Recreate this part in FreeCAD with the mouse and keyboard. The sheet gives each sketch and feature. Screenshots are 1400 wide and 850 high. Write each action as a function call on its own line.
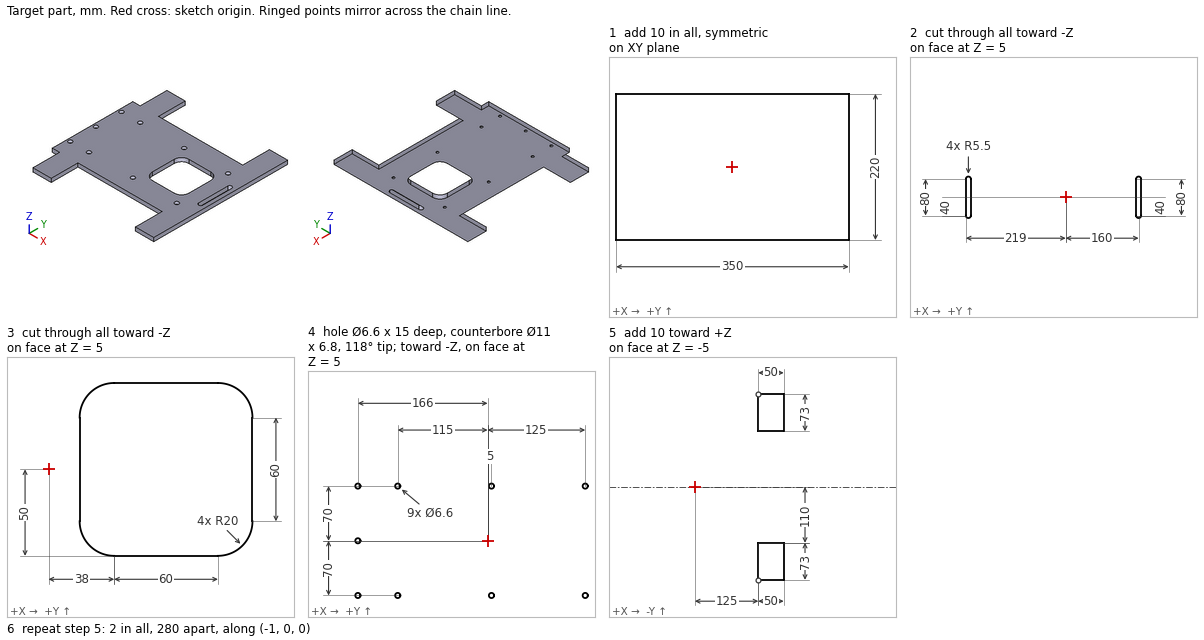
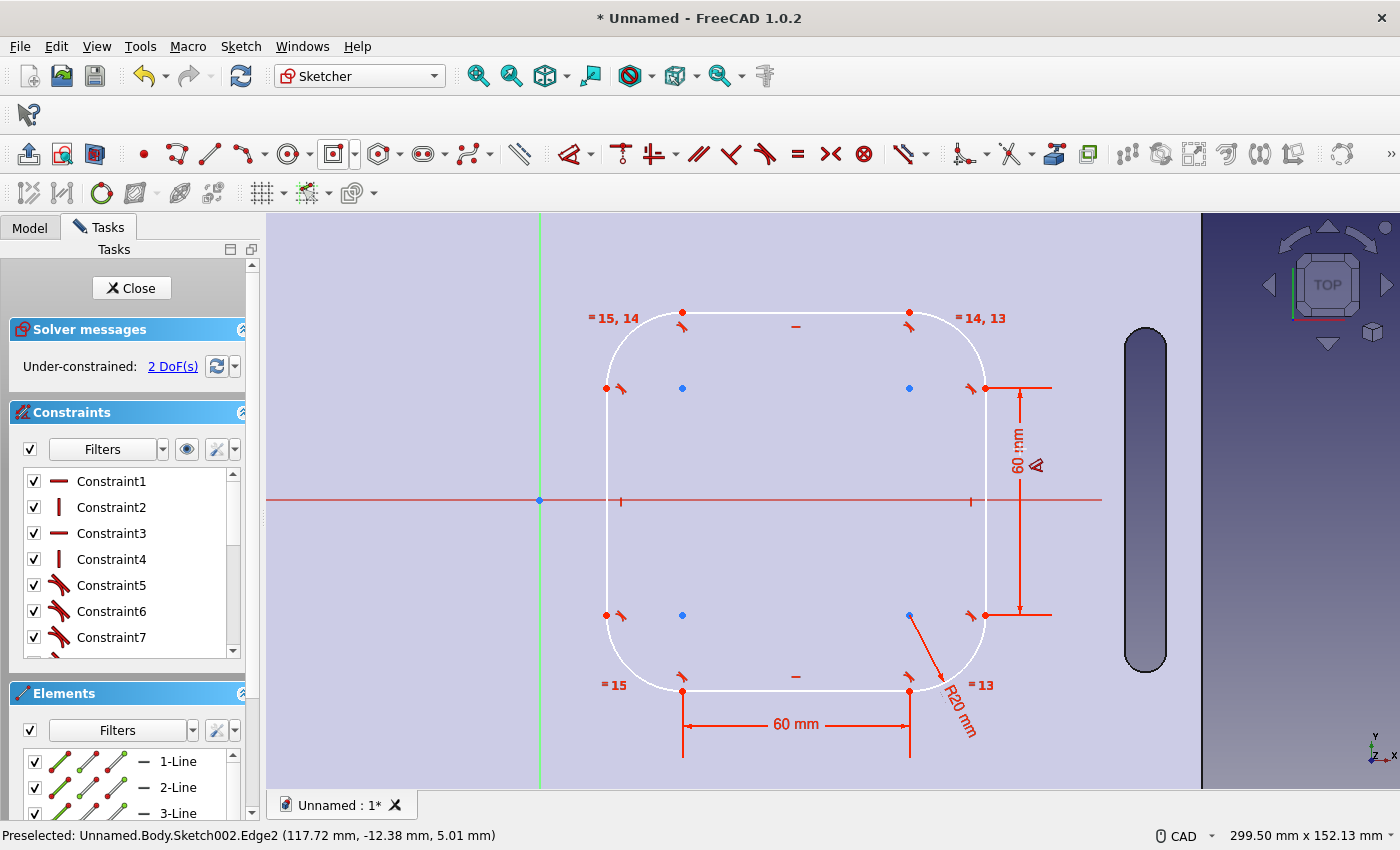
click(683, 691)
click(611, 725)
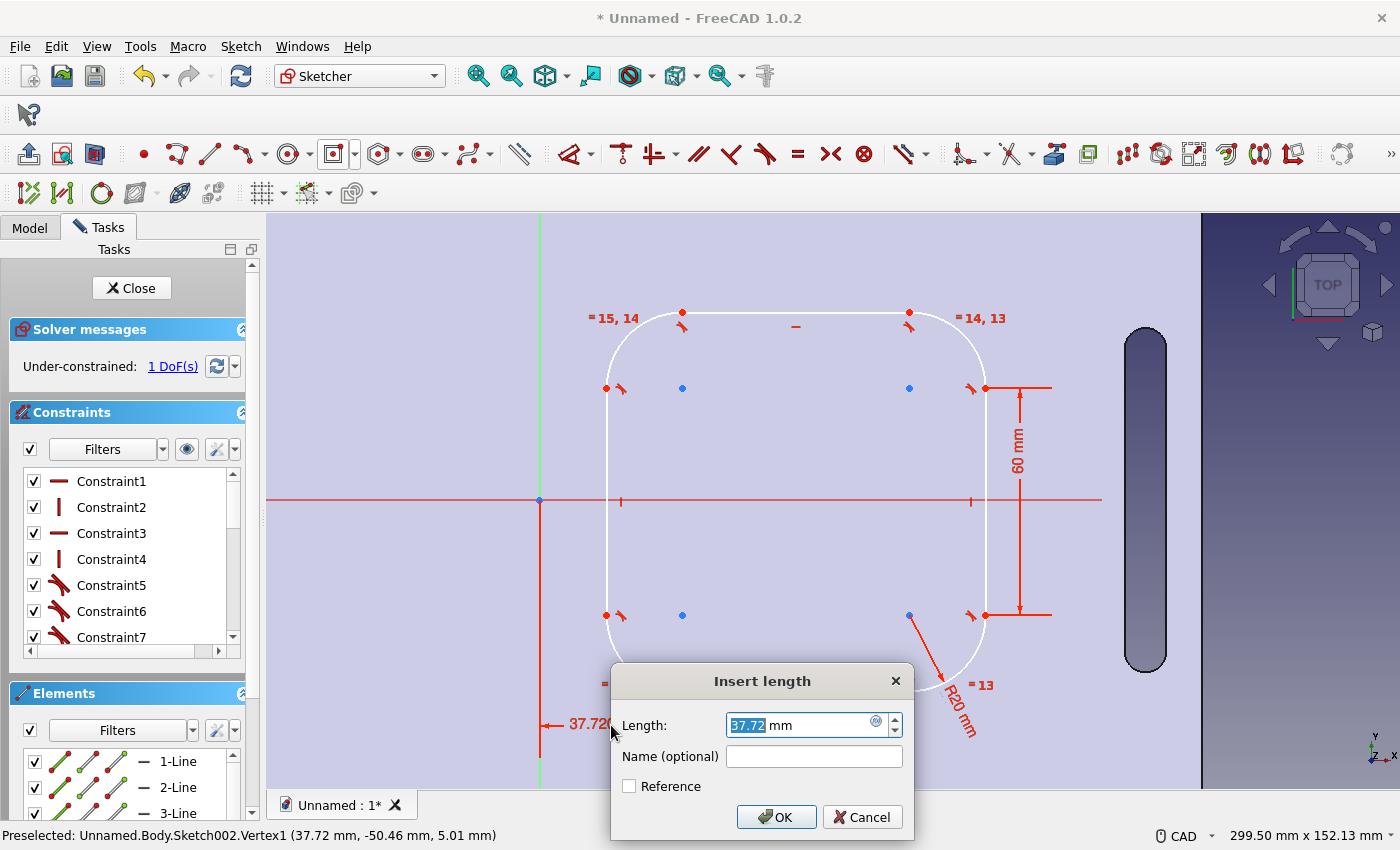
text(38)
key(Return)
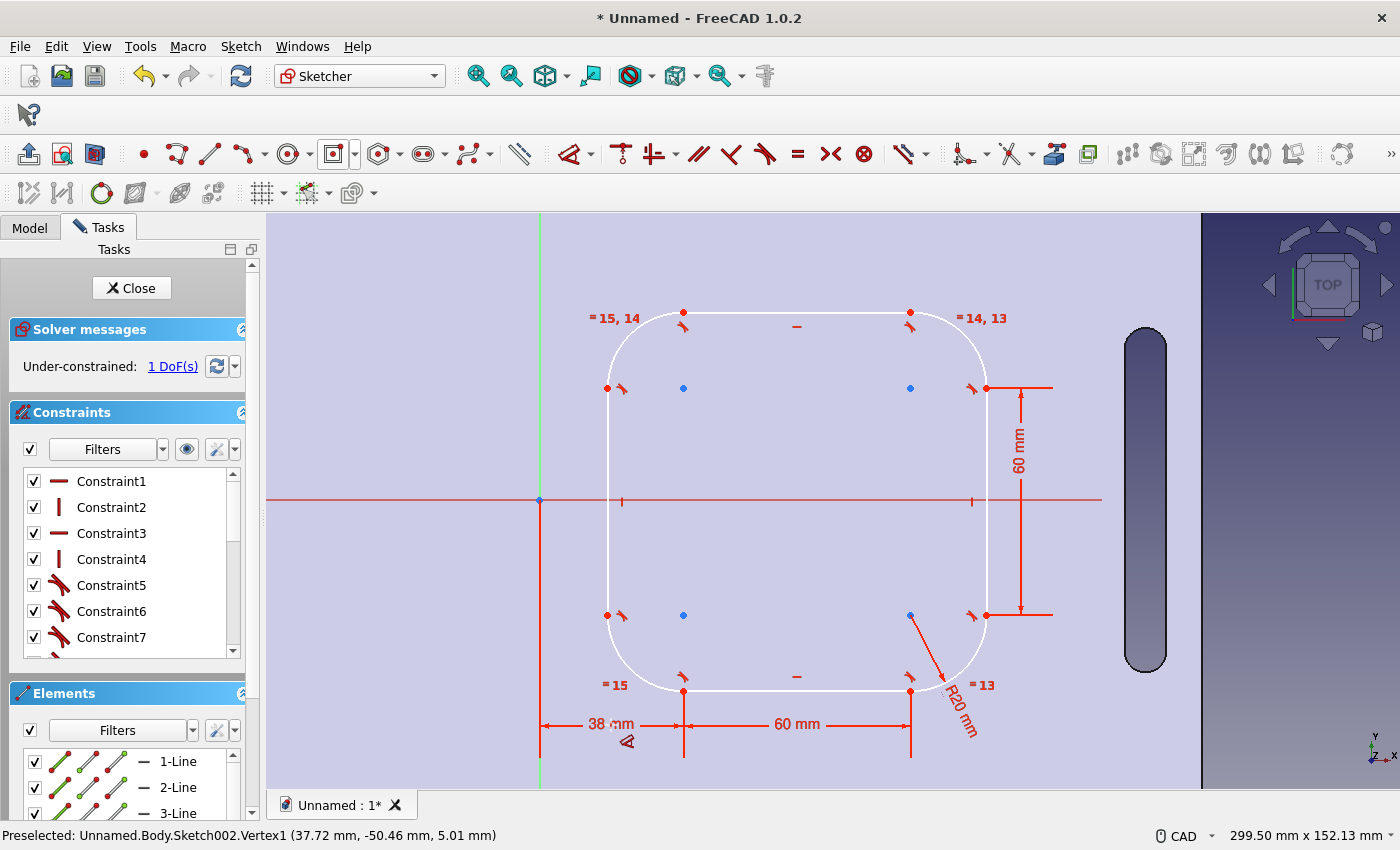
click(684, 691)
click(506, 596)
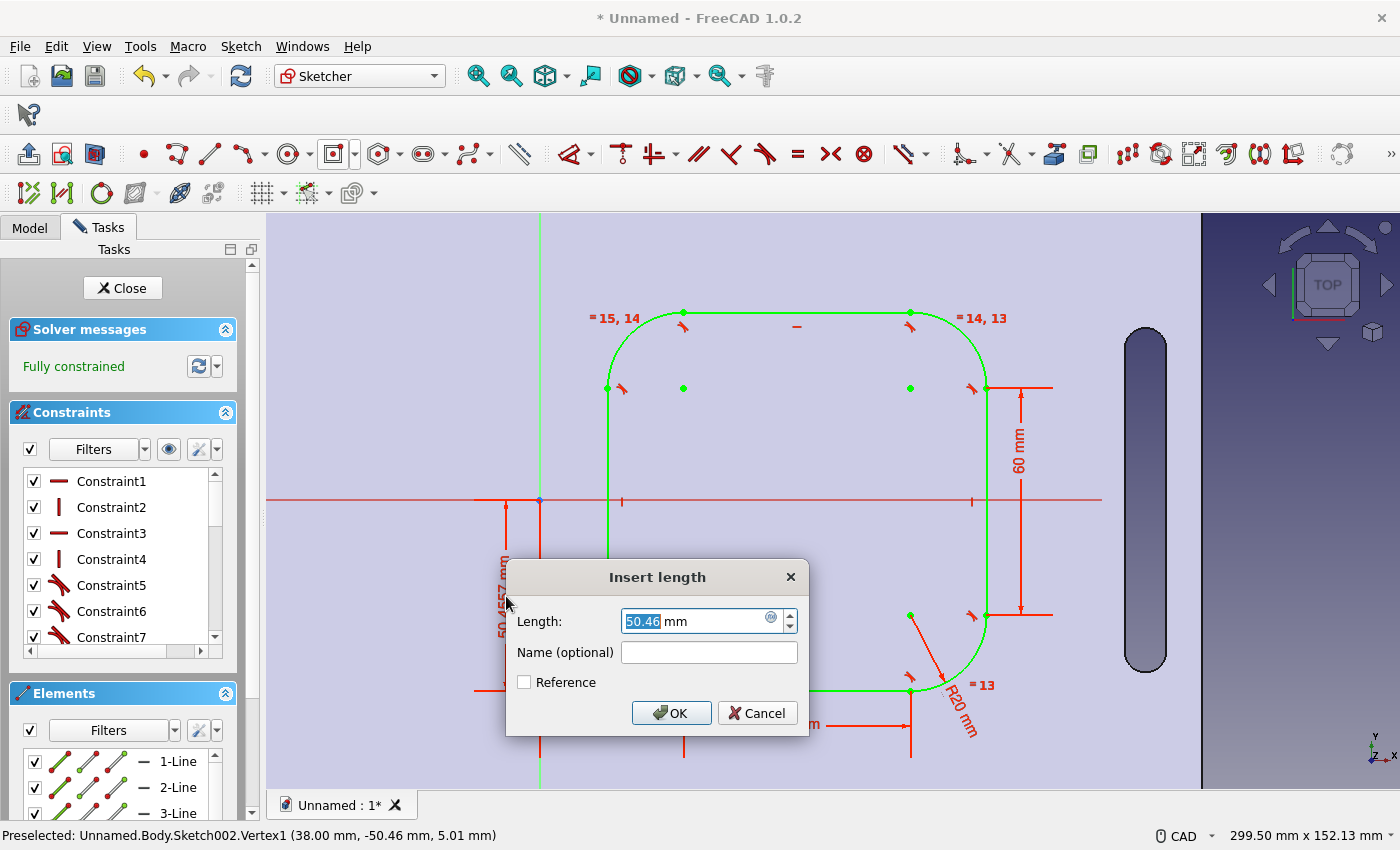
text(50)
key(Return)
key(Escape)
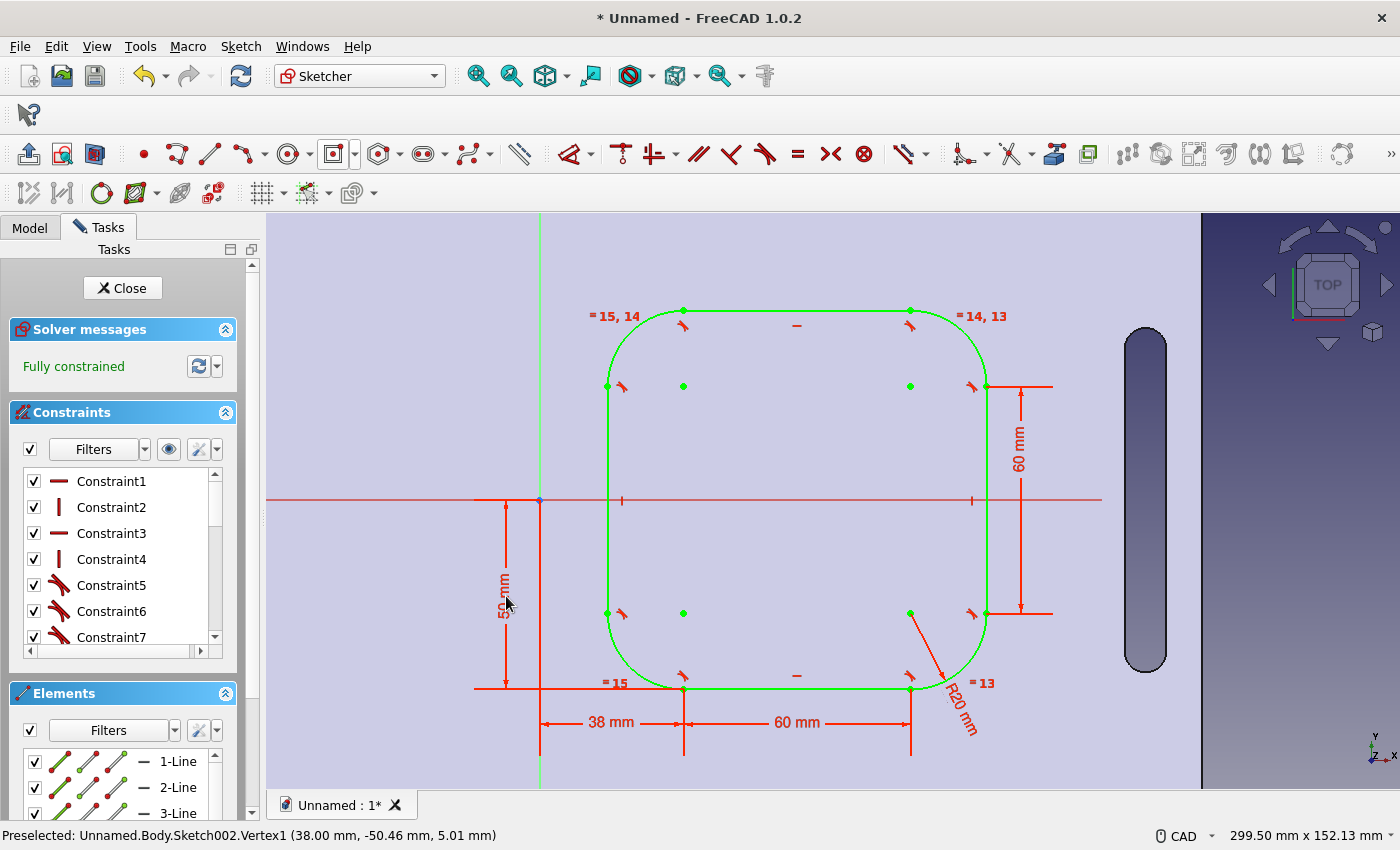
click(123, 288)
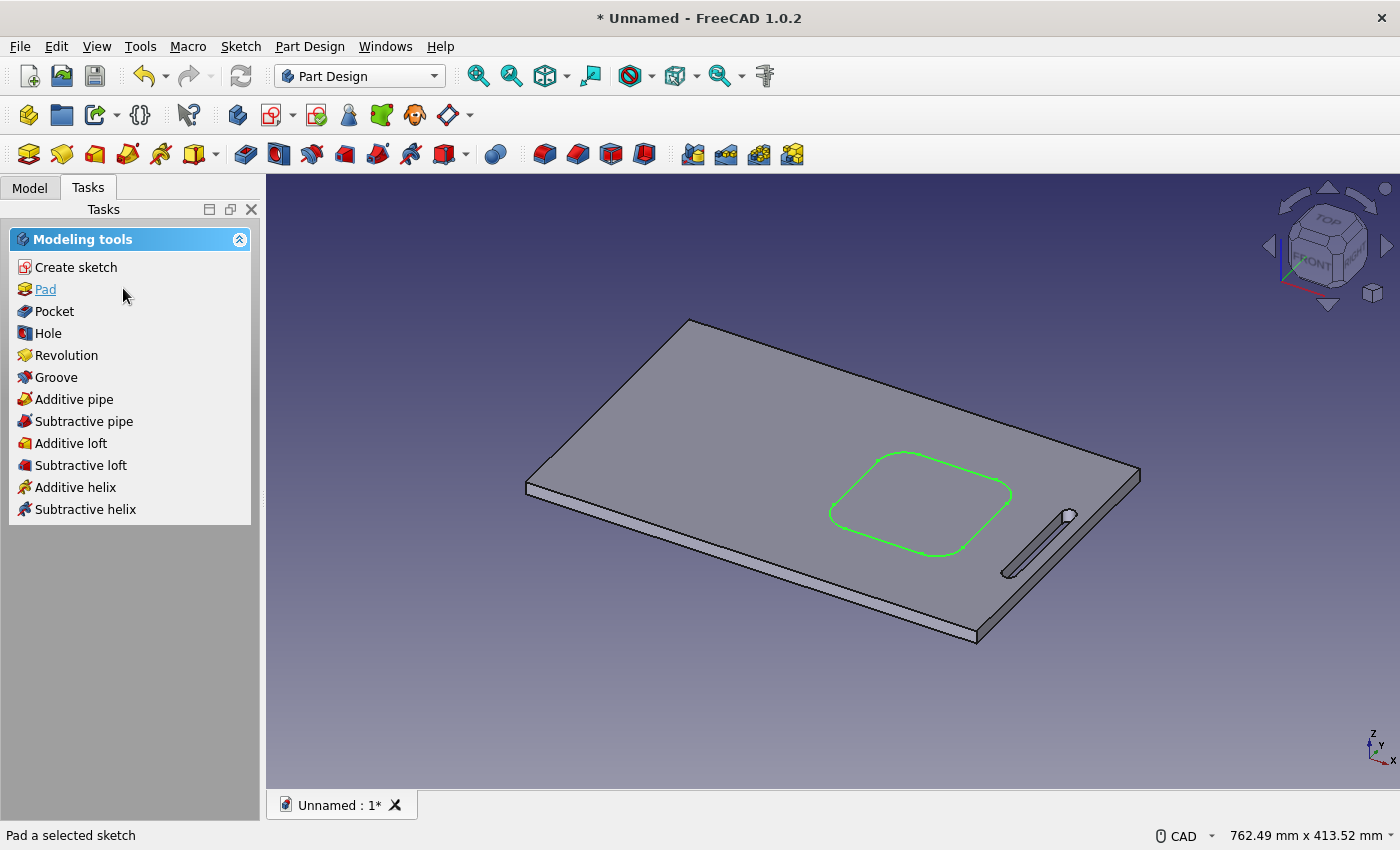
click(246, 154)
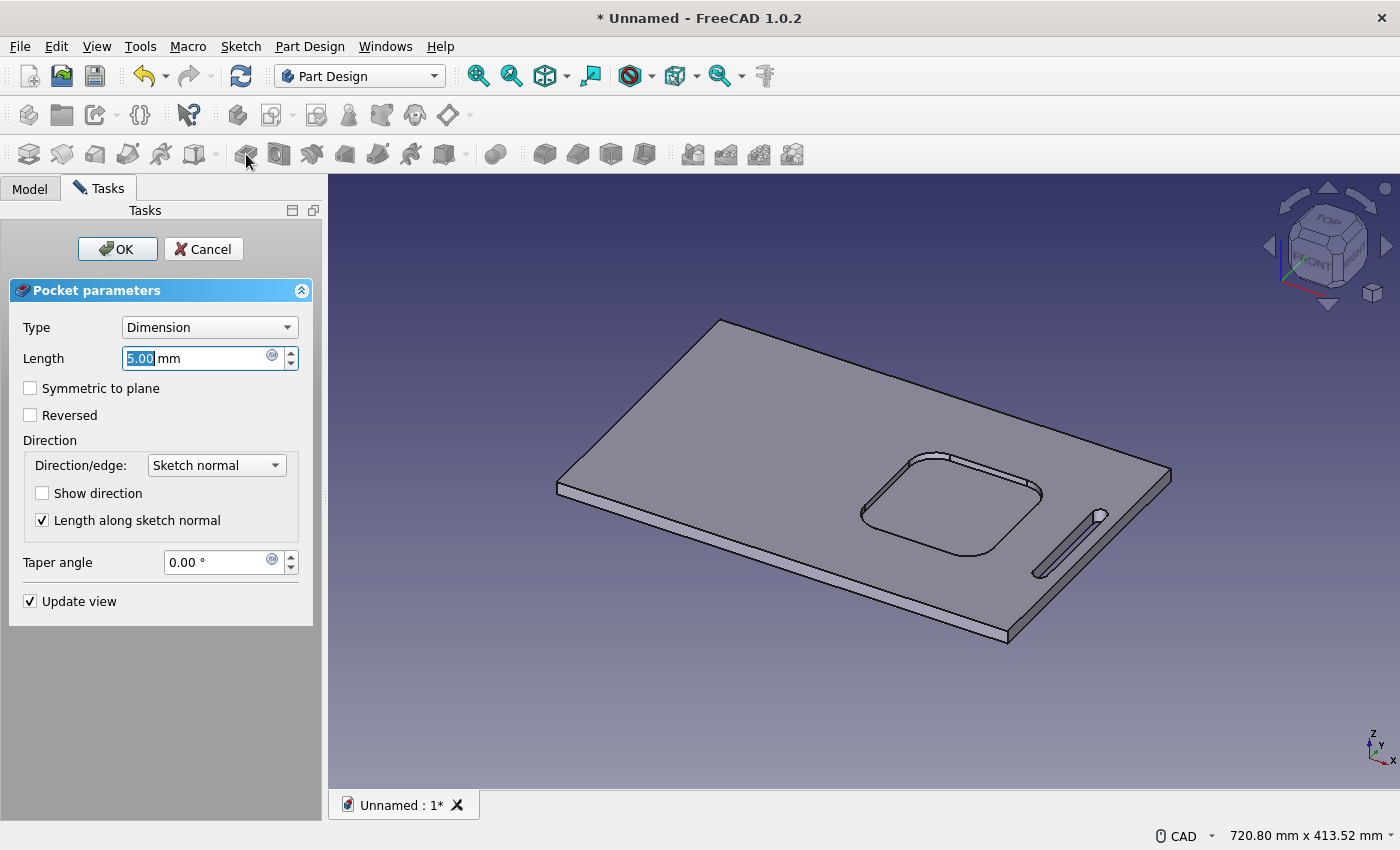
click(210, 328)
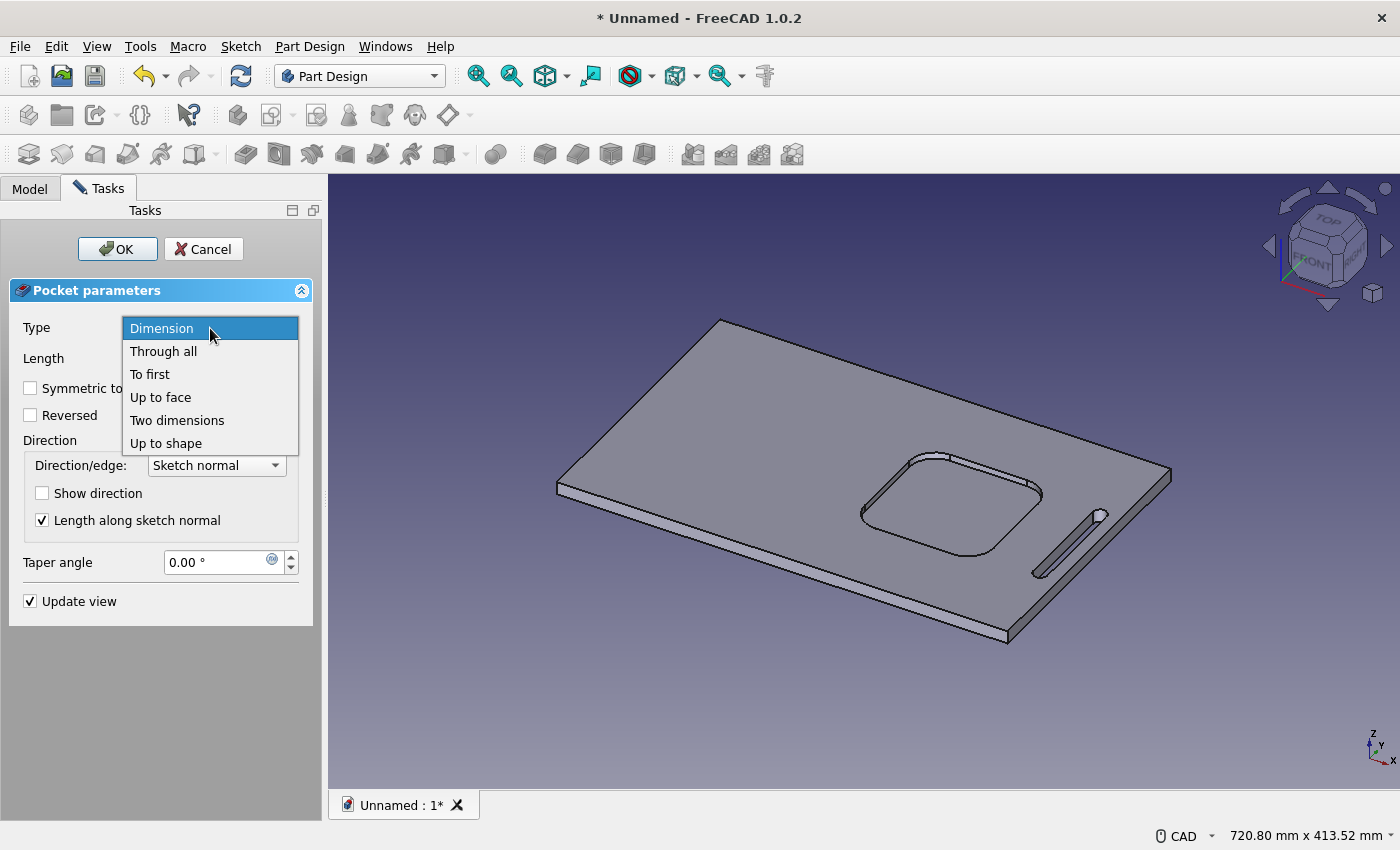
click(208, 352)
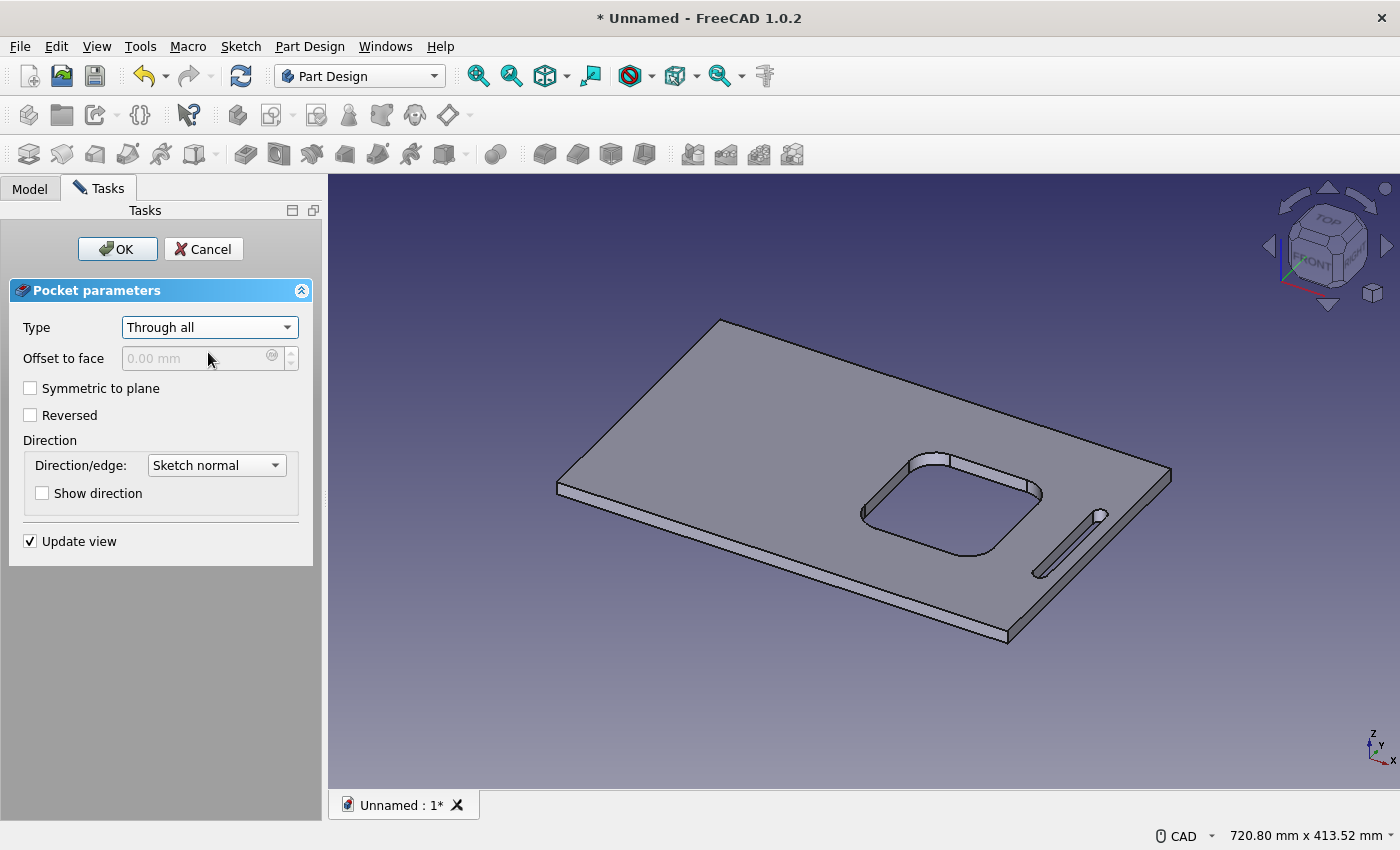
click(118, 249)